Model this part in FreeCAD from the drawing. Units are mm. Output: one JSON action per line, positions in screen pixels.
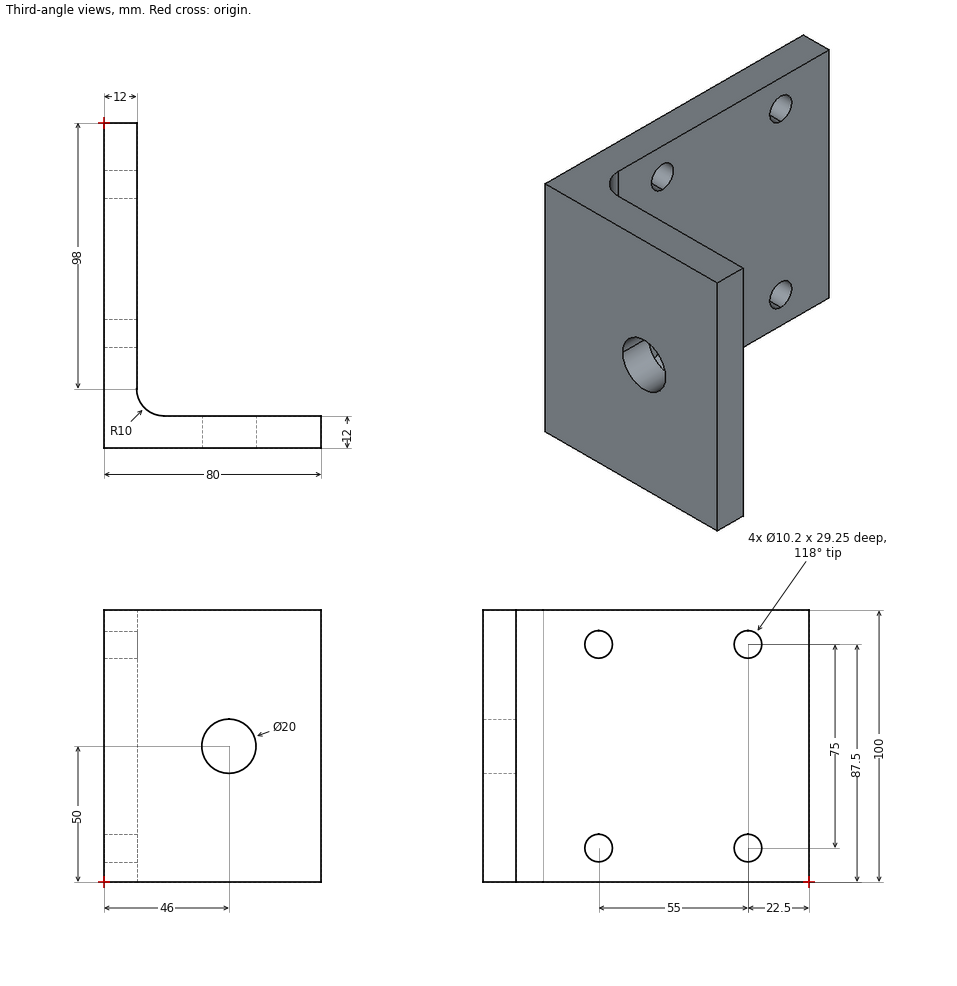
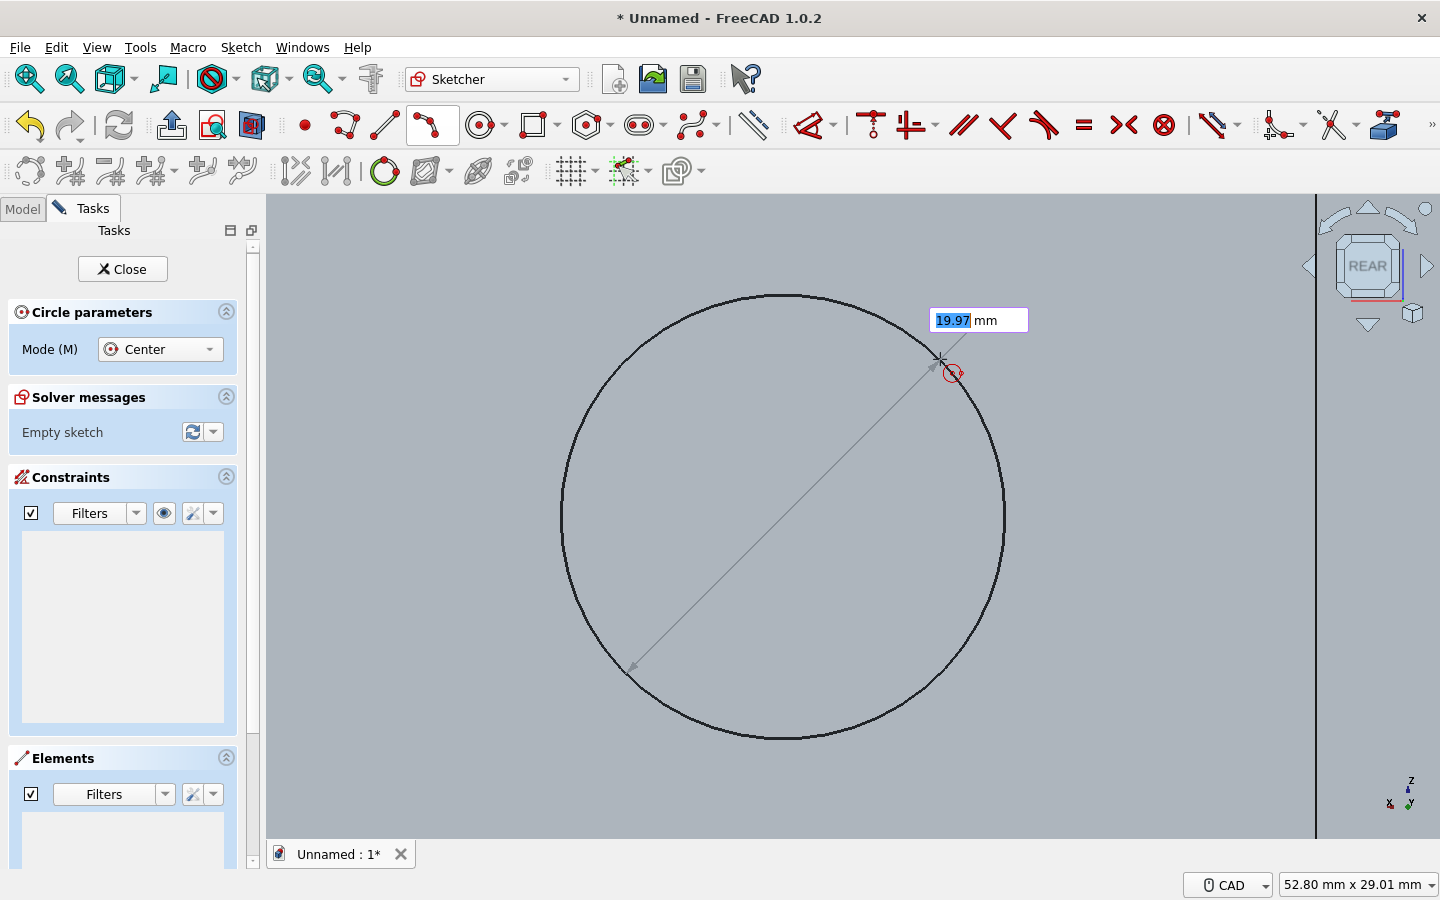
{"action": "type", "text": "20"}
{"action": "key", "text": "Return"}
{"action": "key", "text": "Escape"}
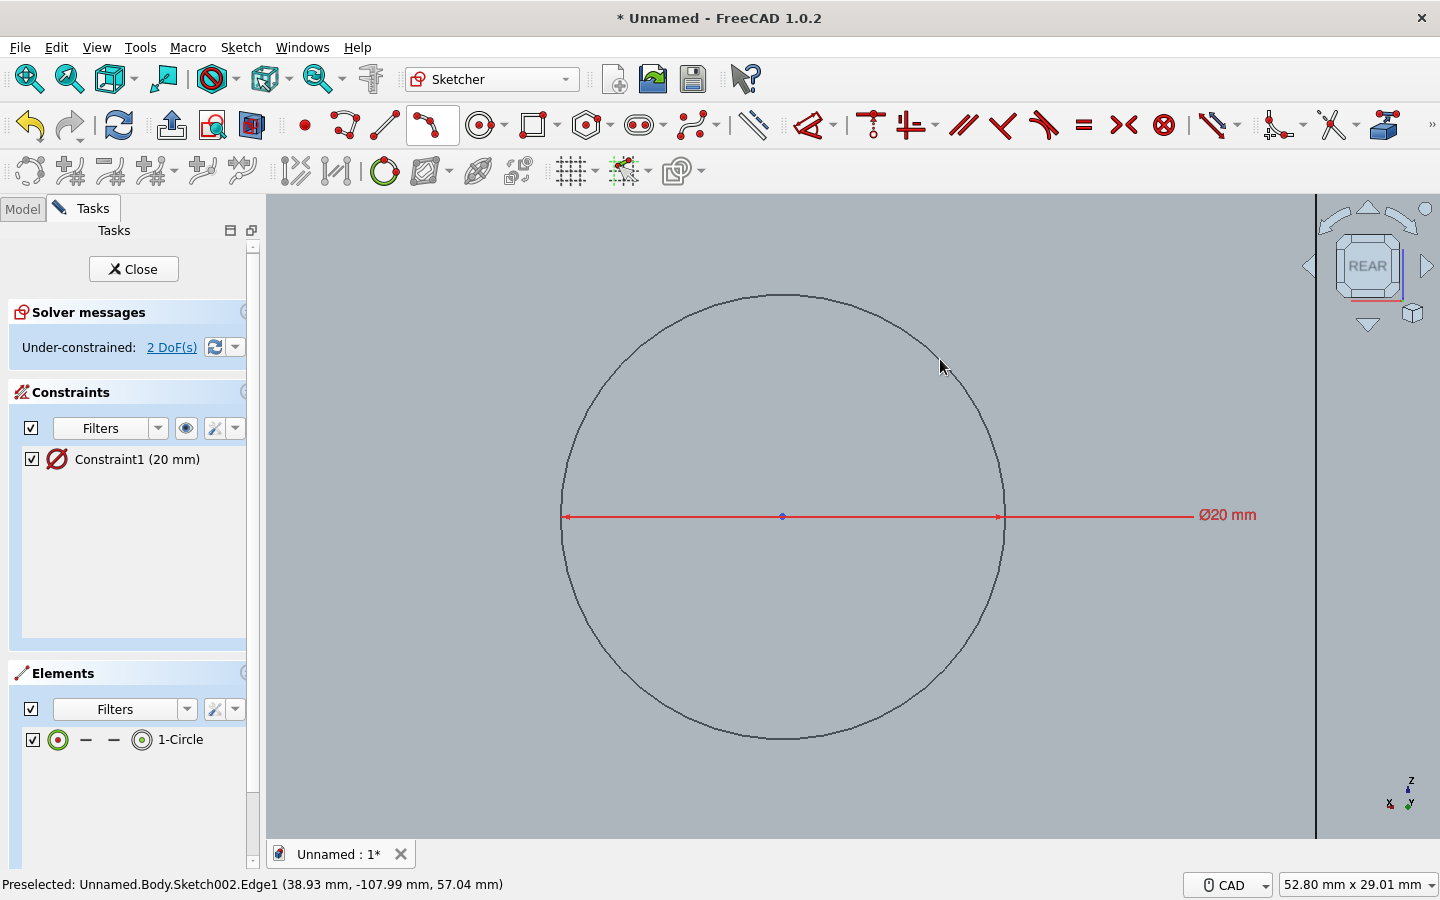
{"action": "left_click", "coordinate": [808, 126]}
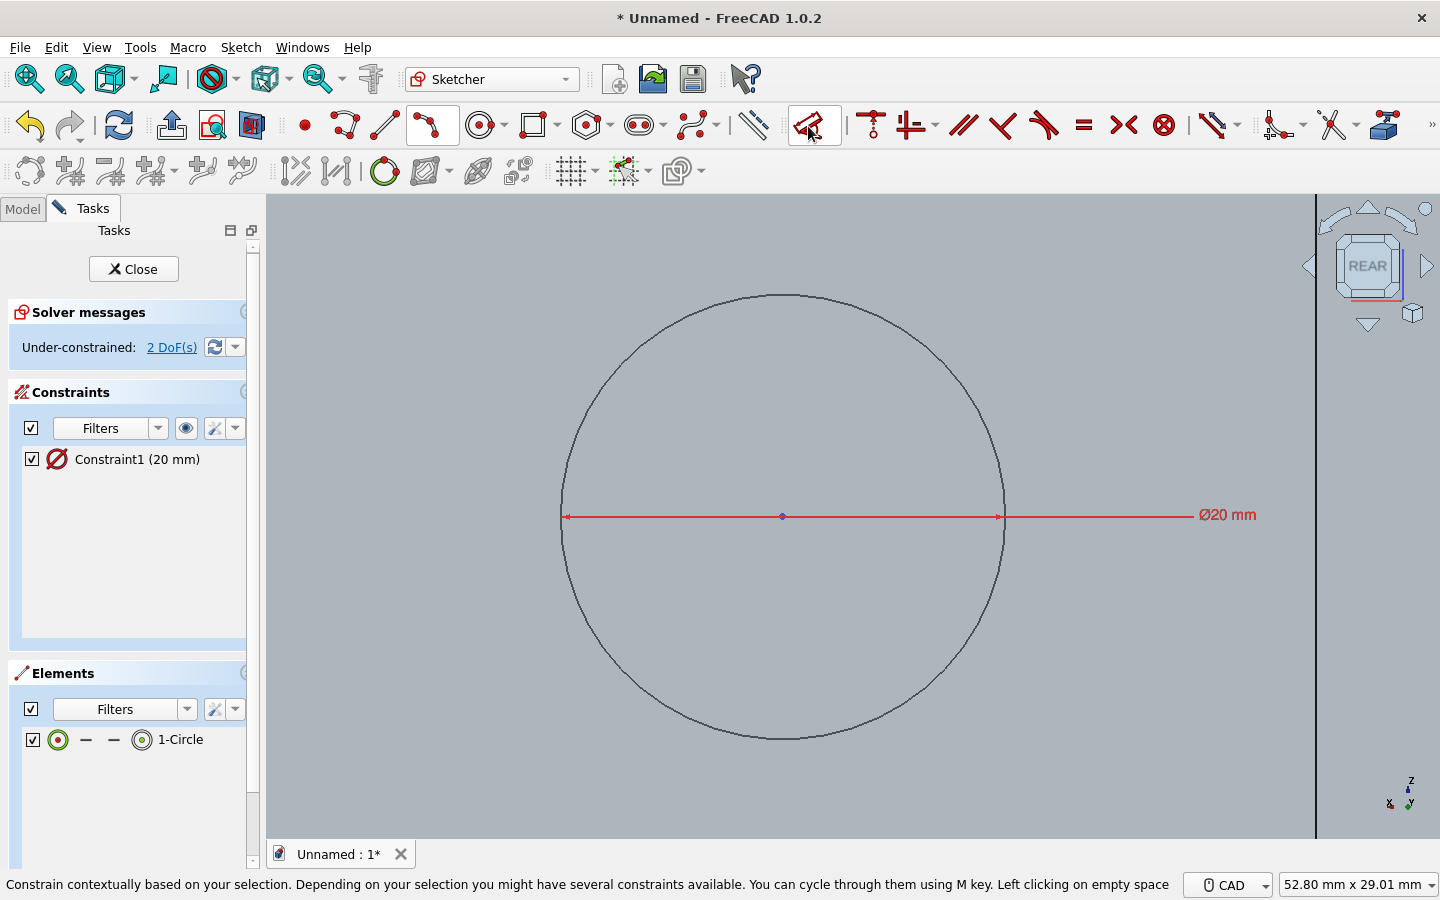
{"action": "left_click", "coordinate": [783, 517]}
{"action": "left_click", "coordinate": [1029, 483]}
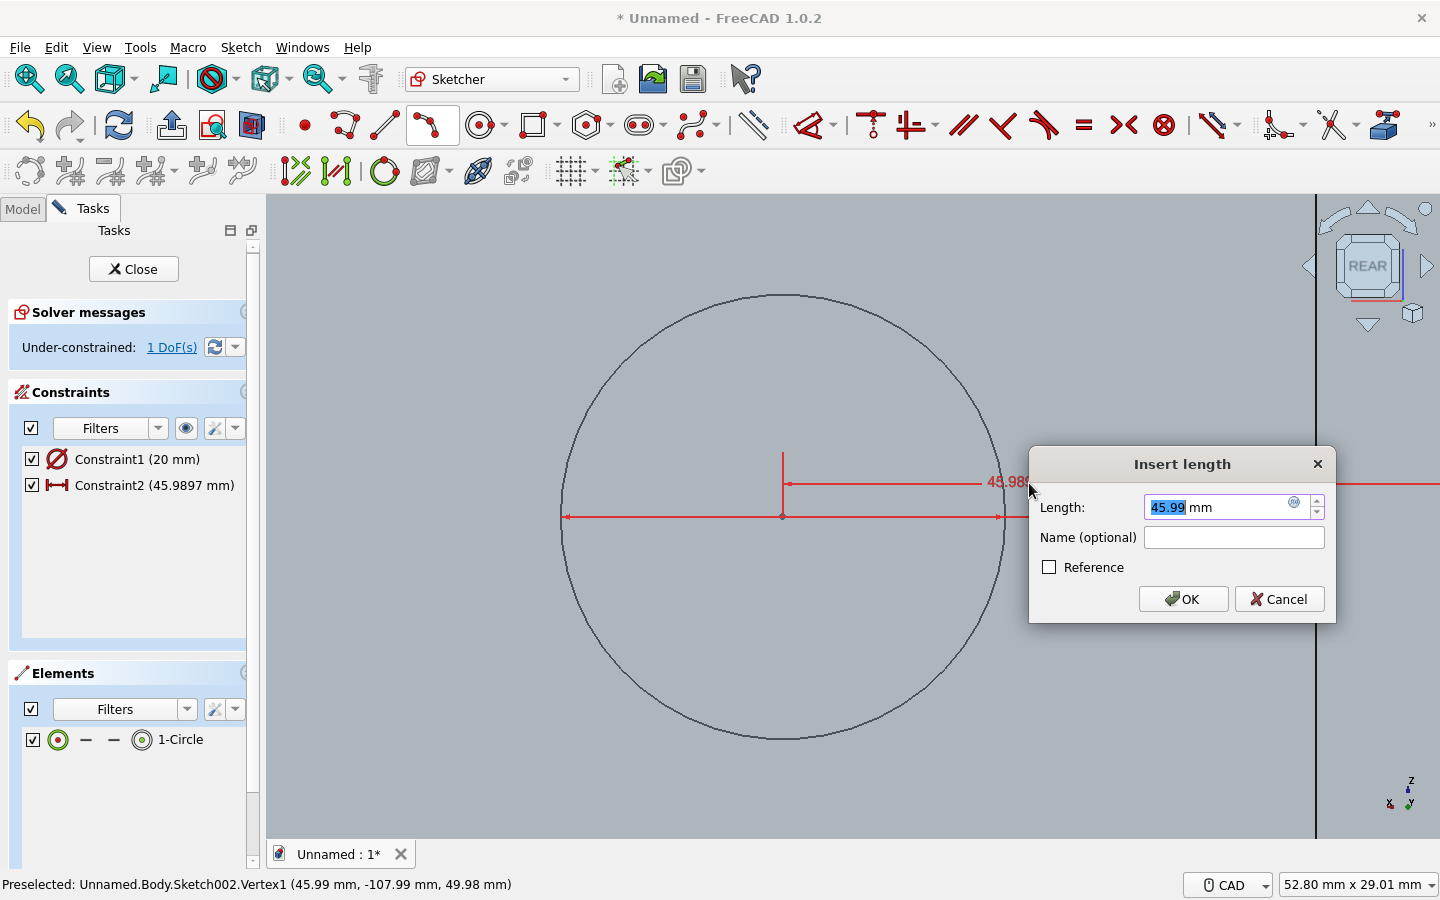
{"action": "type", "text": "46"}
{"action": "key", "text": "Return"}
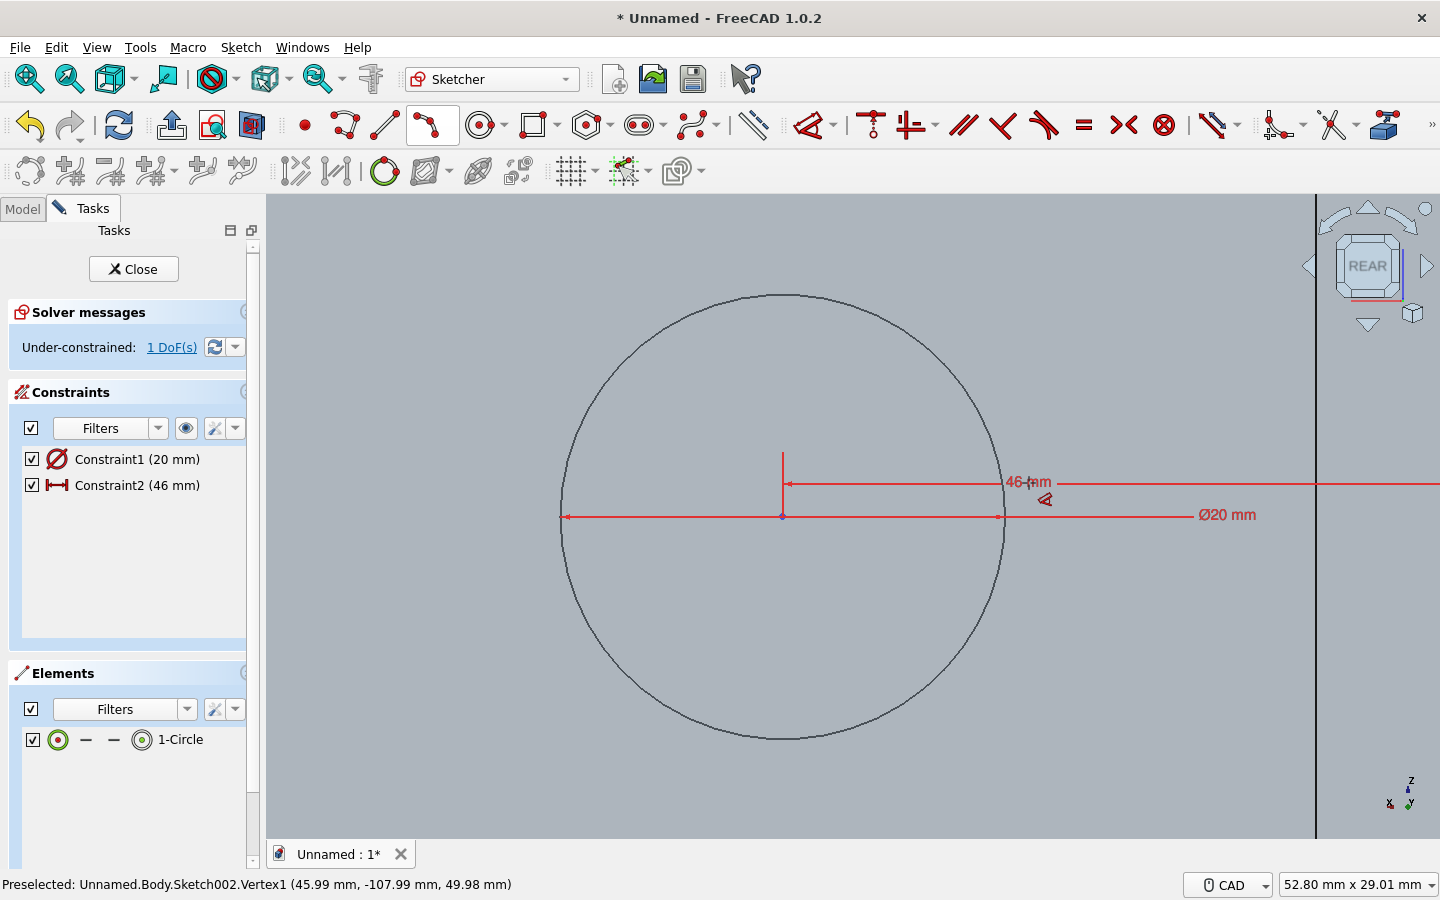
{"action": "left_click", "coordinate": [783, 517]}
{"action": "left_click", "coordinate": [749, 664]}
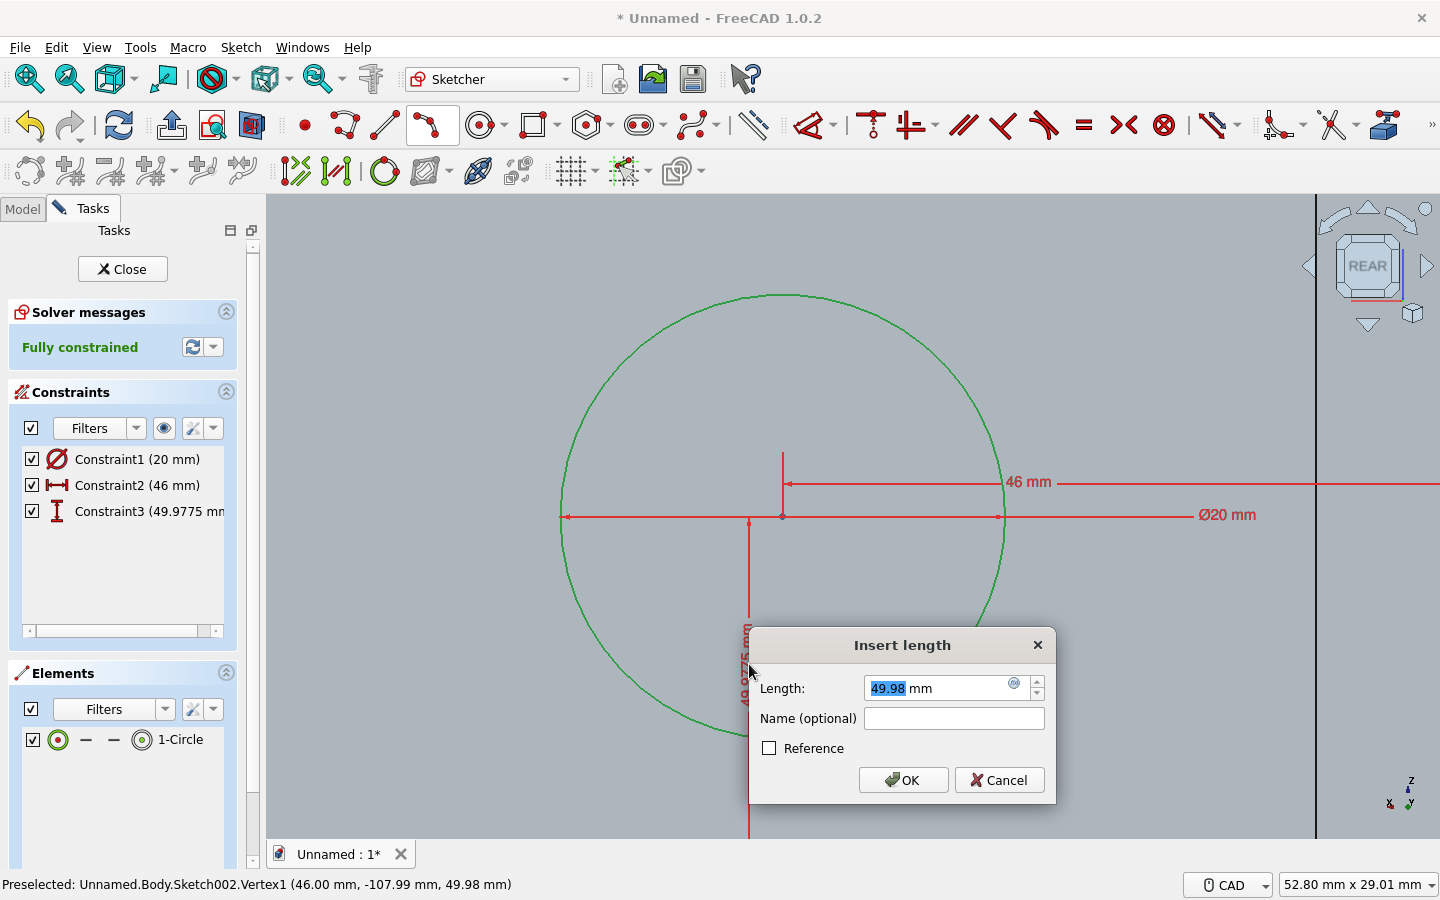
{"action": "type", "text": "50"}
{"action": "key", "text": "Return"}
{"action": "key", "text": "Escape"}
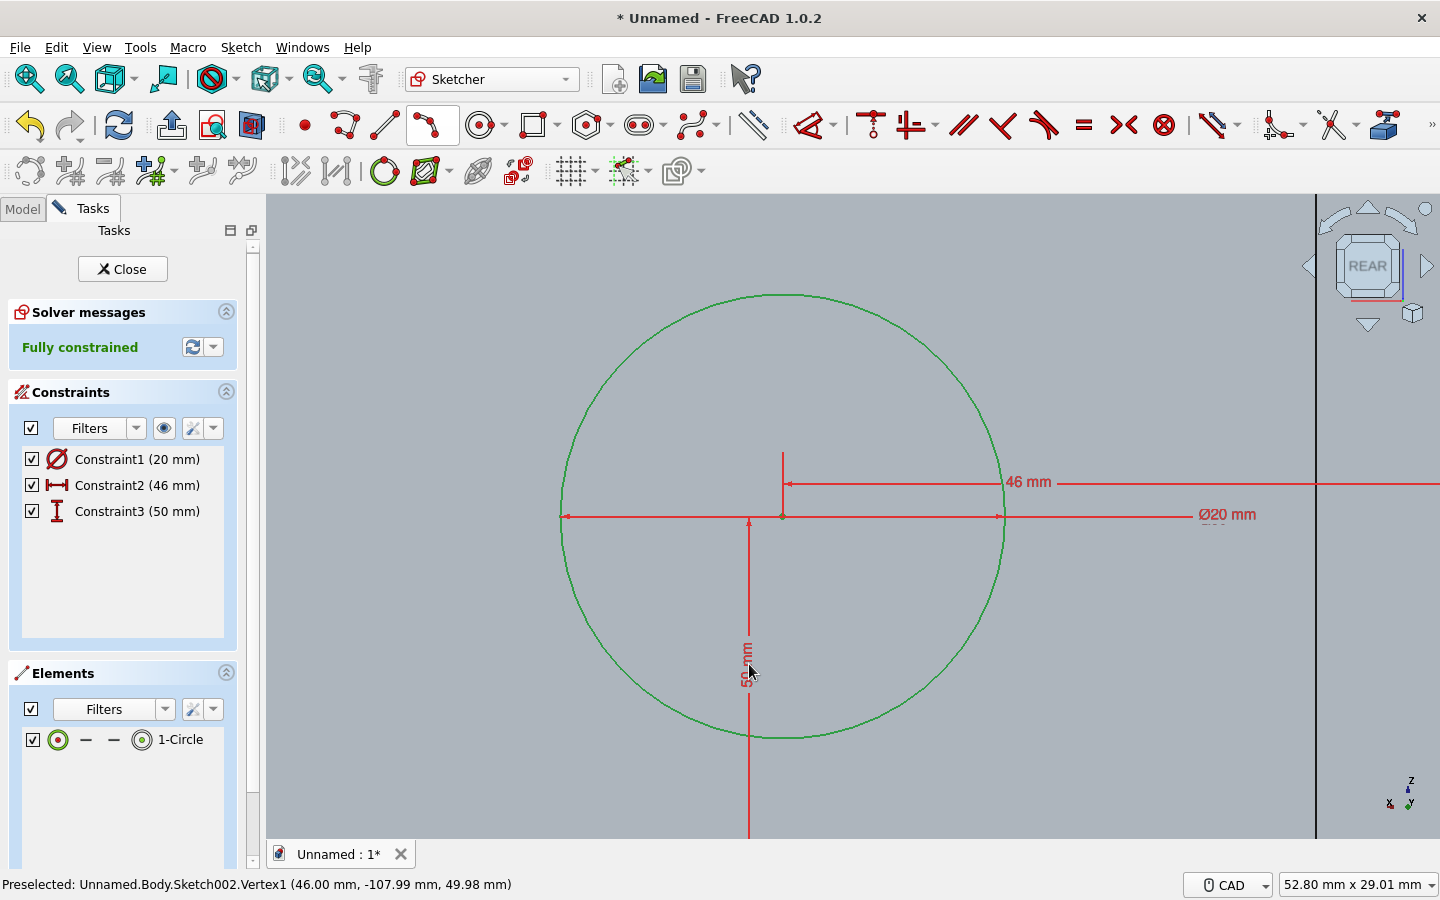
{"action": "left_click", "coordinate": [123, 269]}